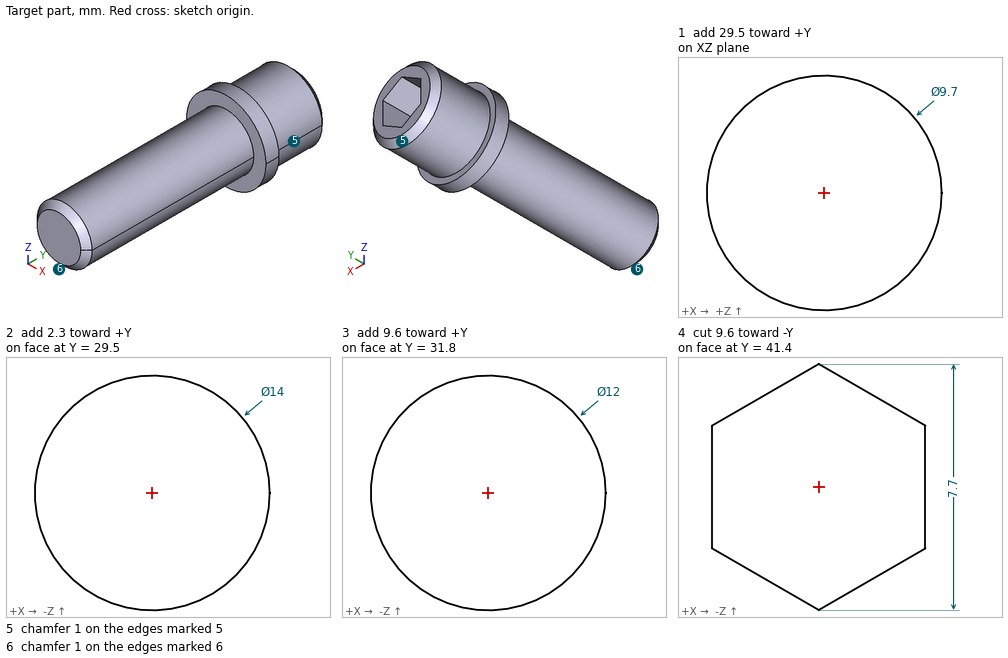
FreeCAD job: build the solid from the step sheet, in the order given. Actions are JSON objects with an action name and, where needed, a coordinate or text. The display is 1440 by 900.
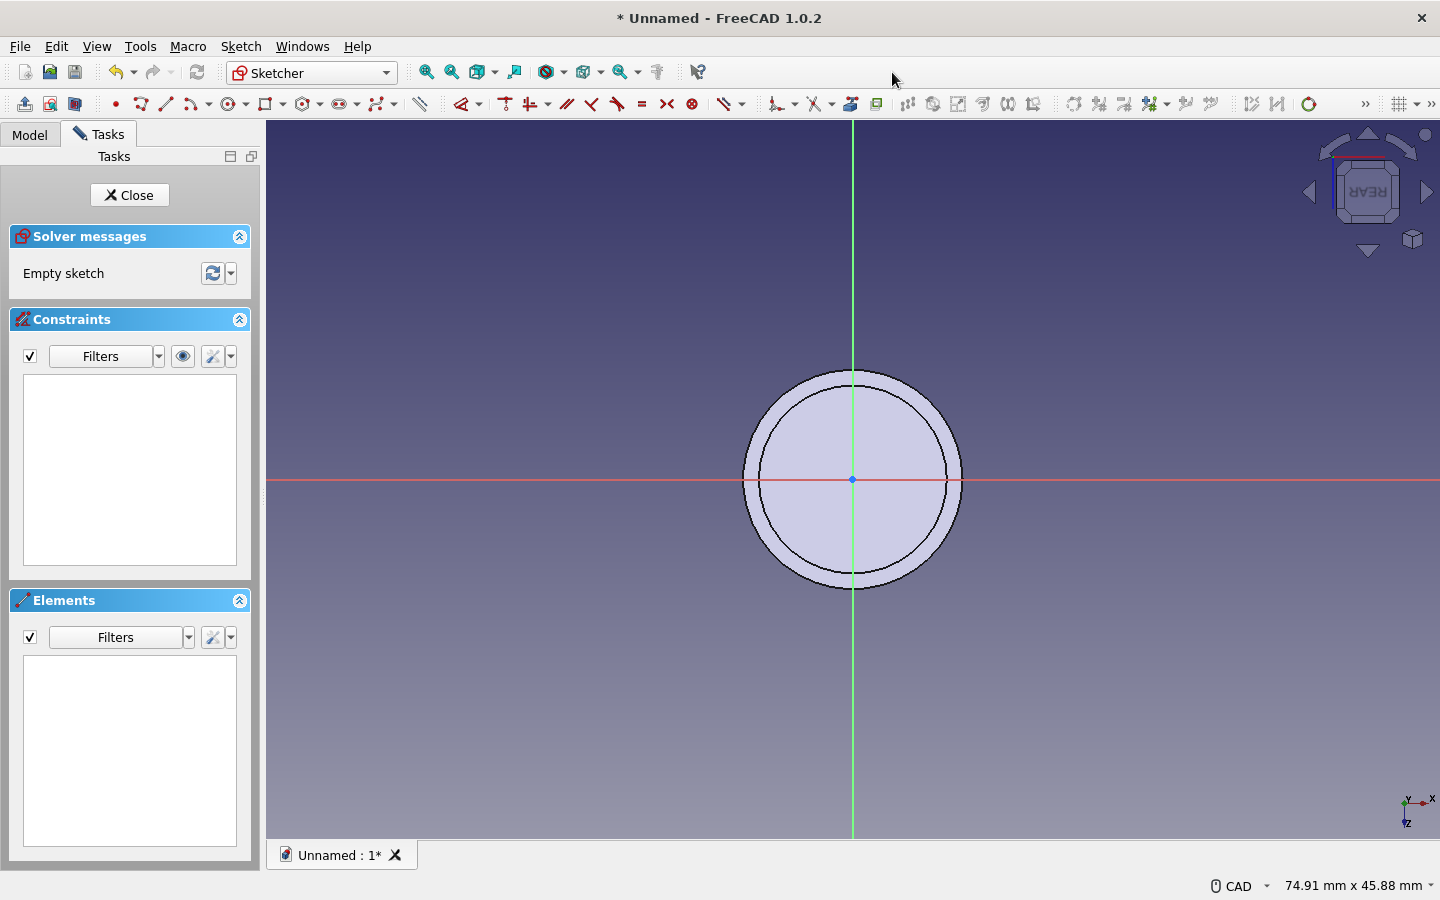
{"action": "scroll", "coordinate": [875, 479], "scroll_direction": "up", "scroll_amount": 7}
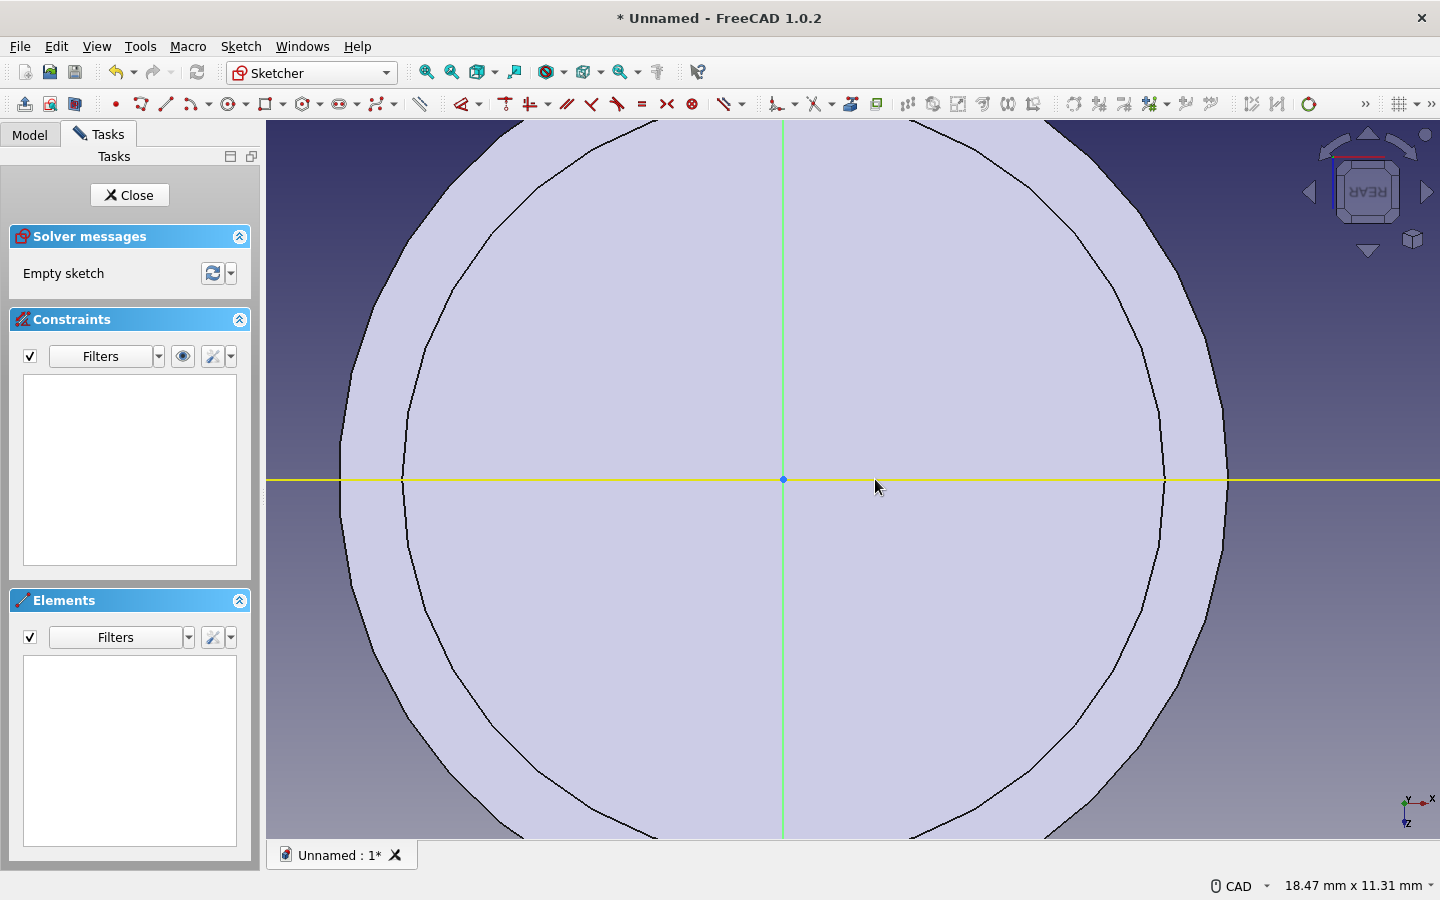
{"action": "left_click", "coordinate": [302, 104]}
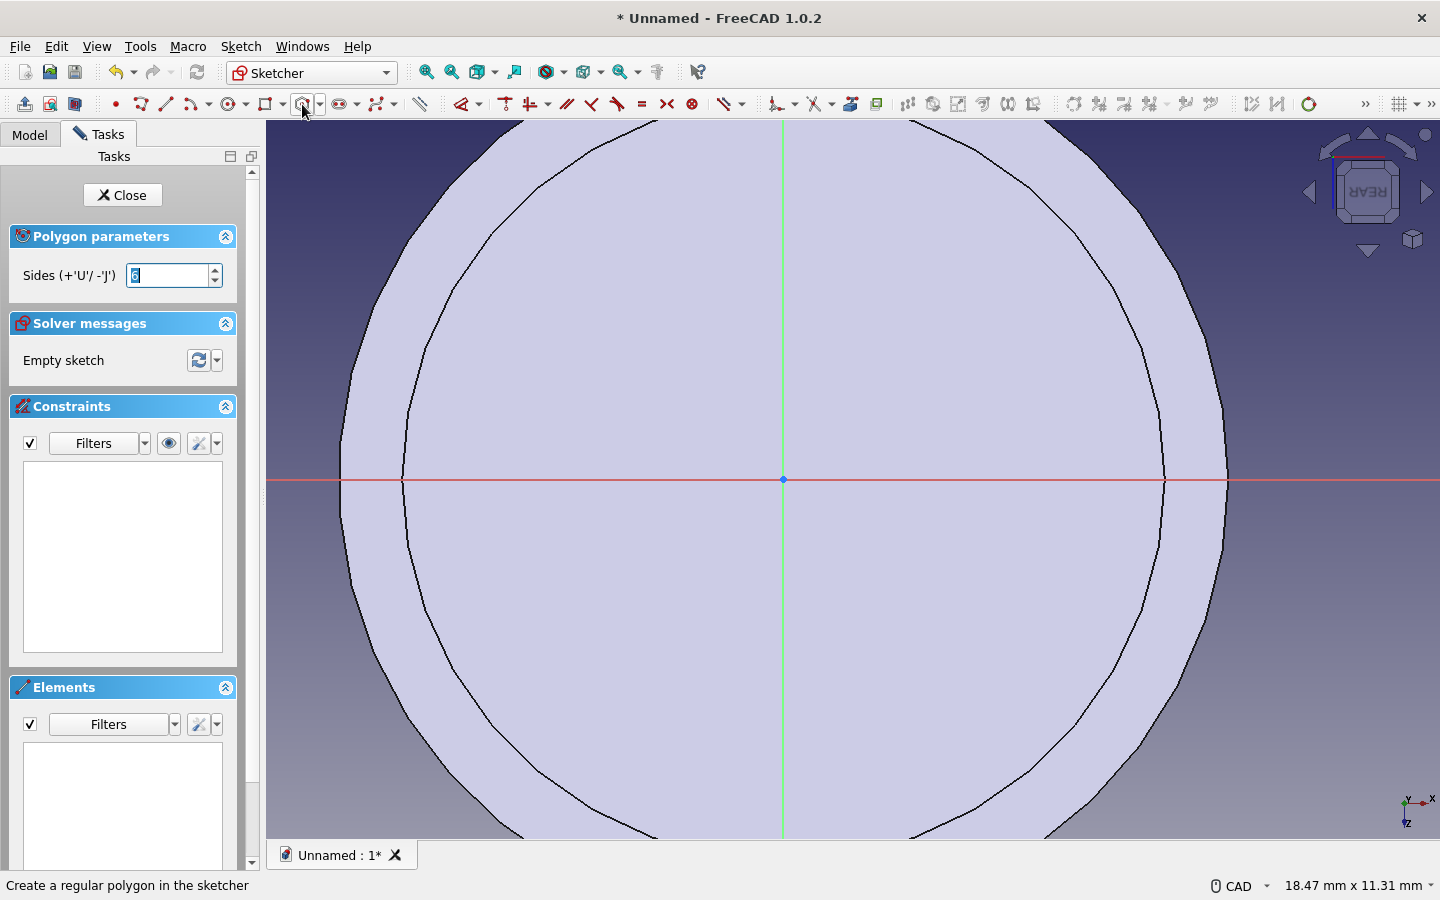
{"action": "left_click", "coordinate": [783, 479]}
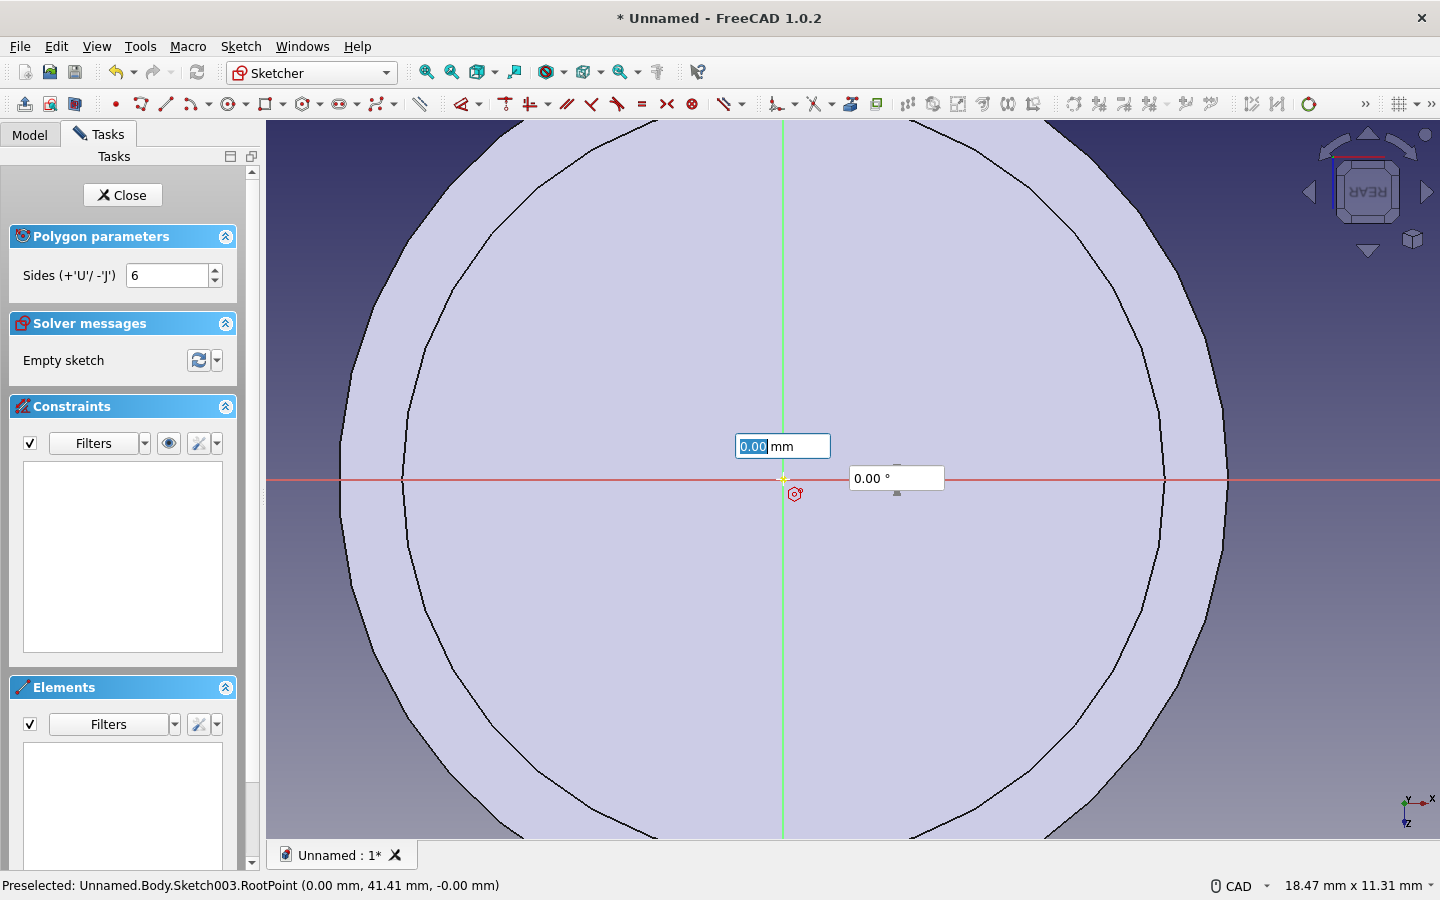
{"action": "left_click", "coordinate": [783, 235]}
{"action": "right_click", "coordinate": [783, 235]}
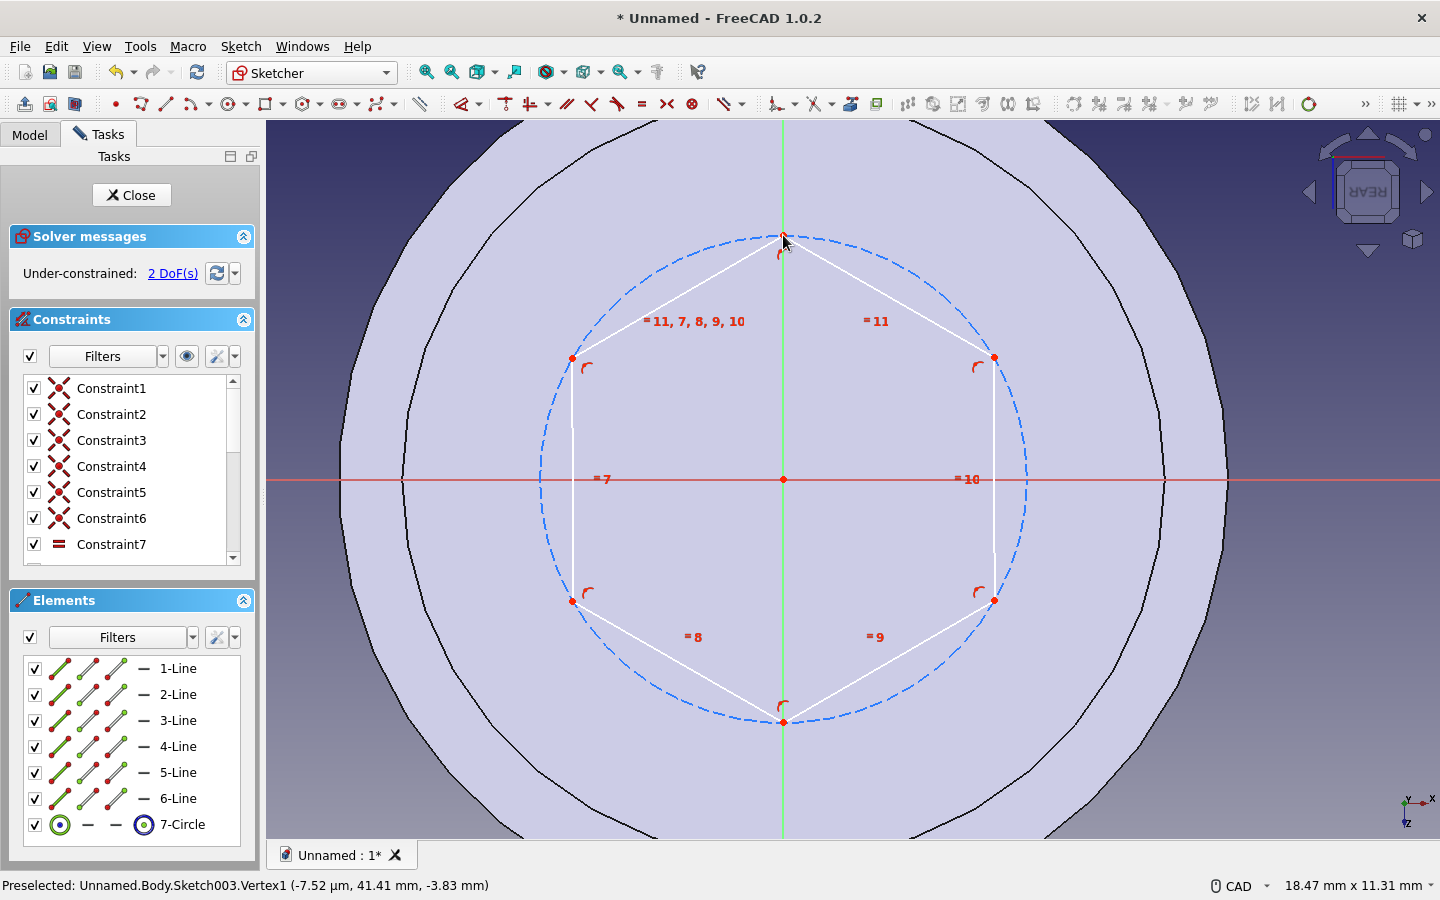
{"action": "left_click", "coordinate": [573, 431]}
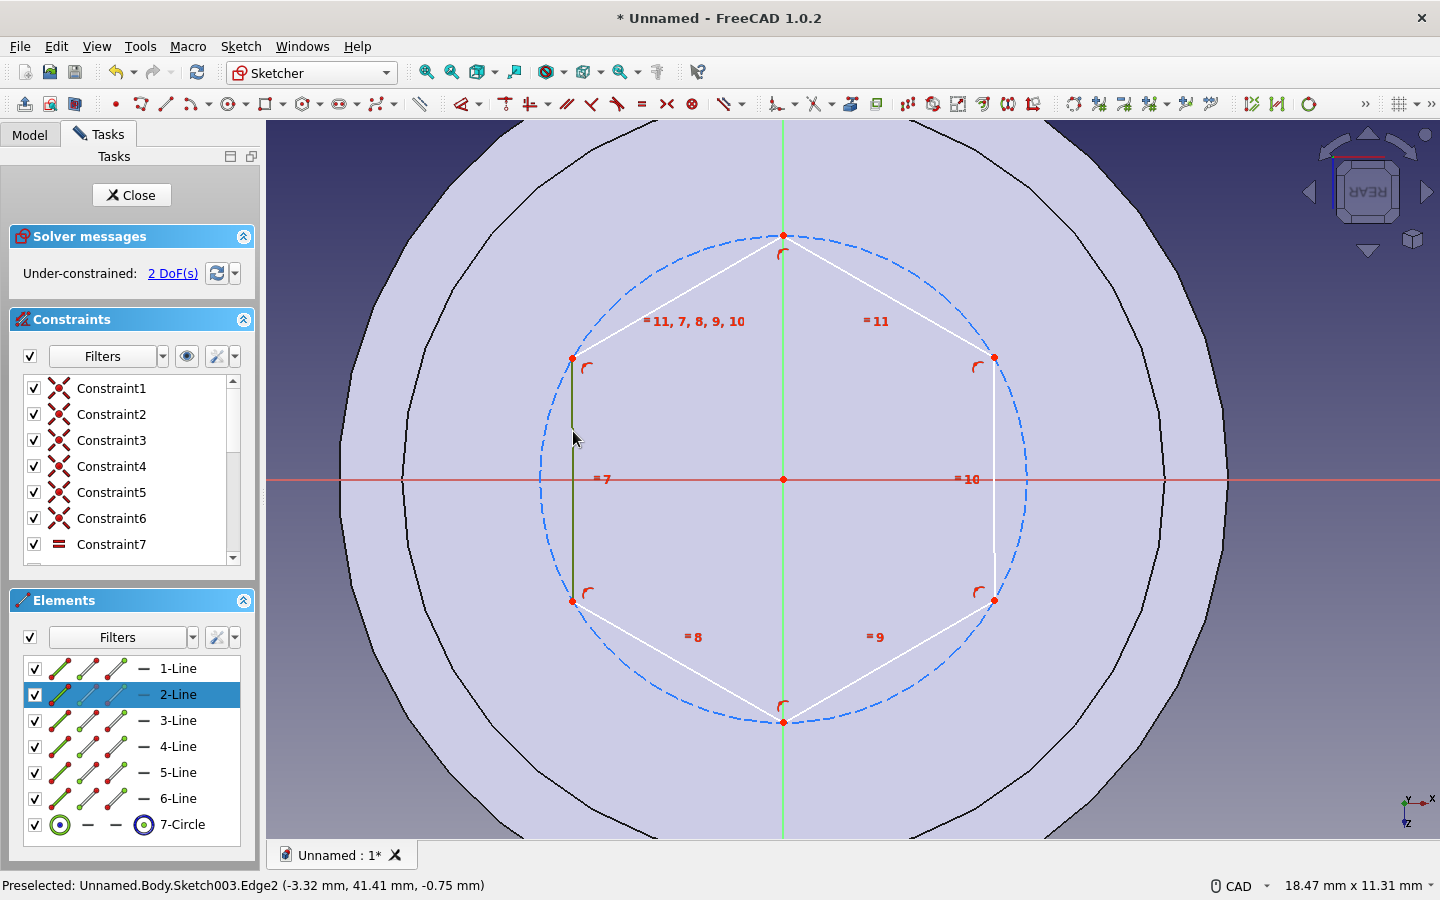
{"action": "left_click", "coordinate": [548, 104]}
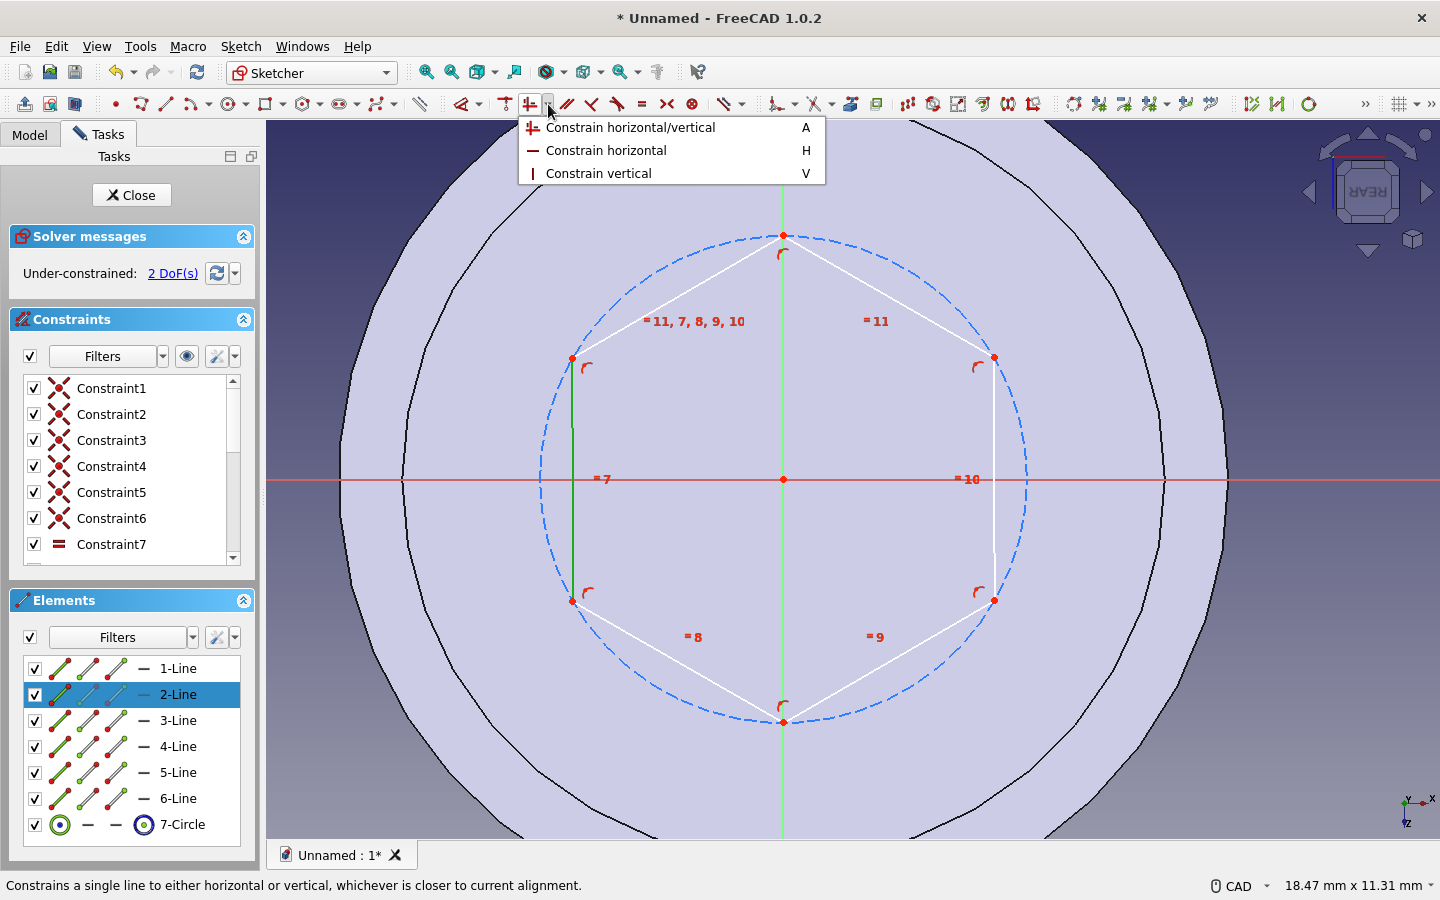
{"action": "left_click", "coordinate": [672, 174]}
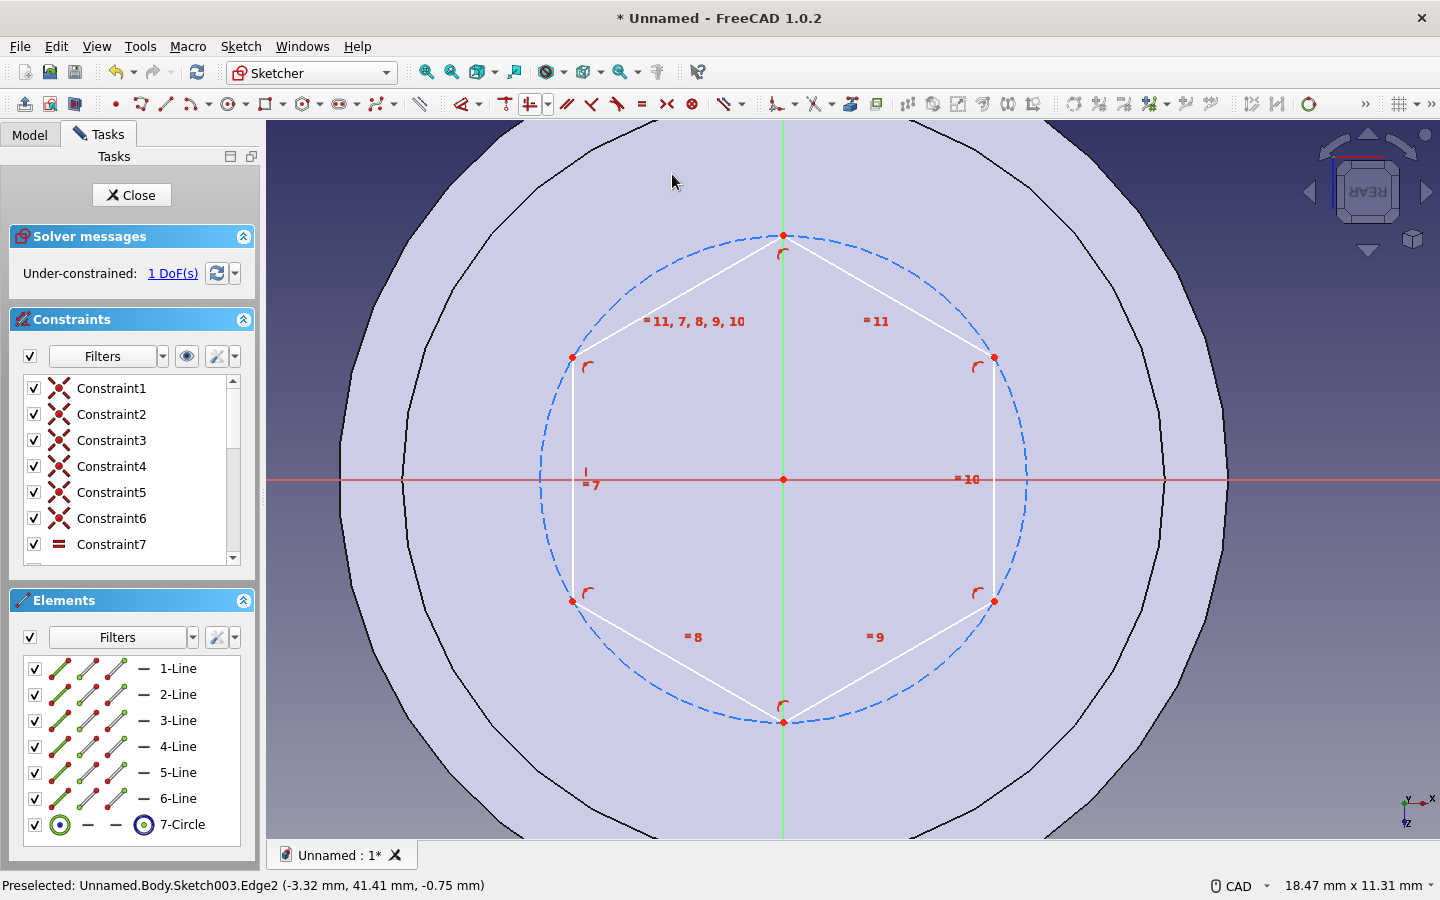
{"action": "left_click", "coordinate": [460, 104]}